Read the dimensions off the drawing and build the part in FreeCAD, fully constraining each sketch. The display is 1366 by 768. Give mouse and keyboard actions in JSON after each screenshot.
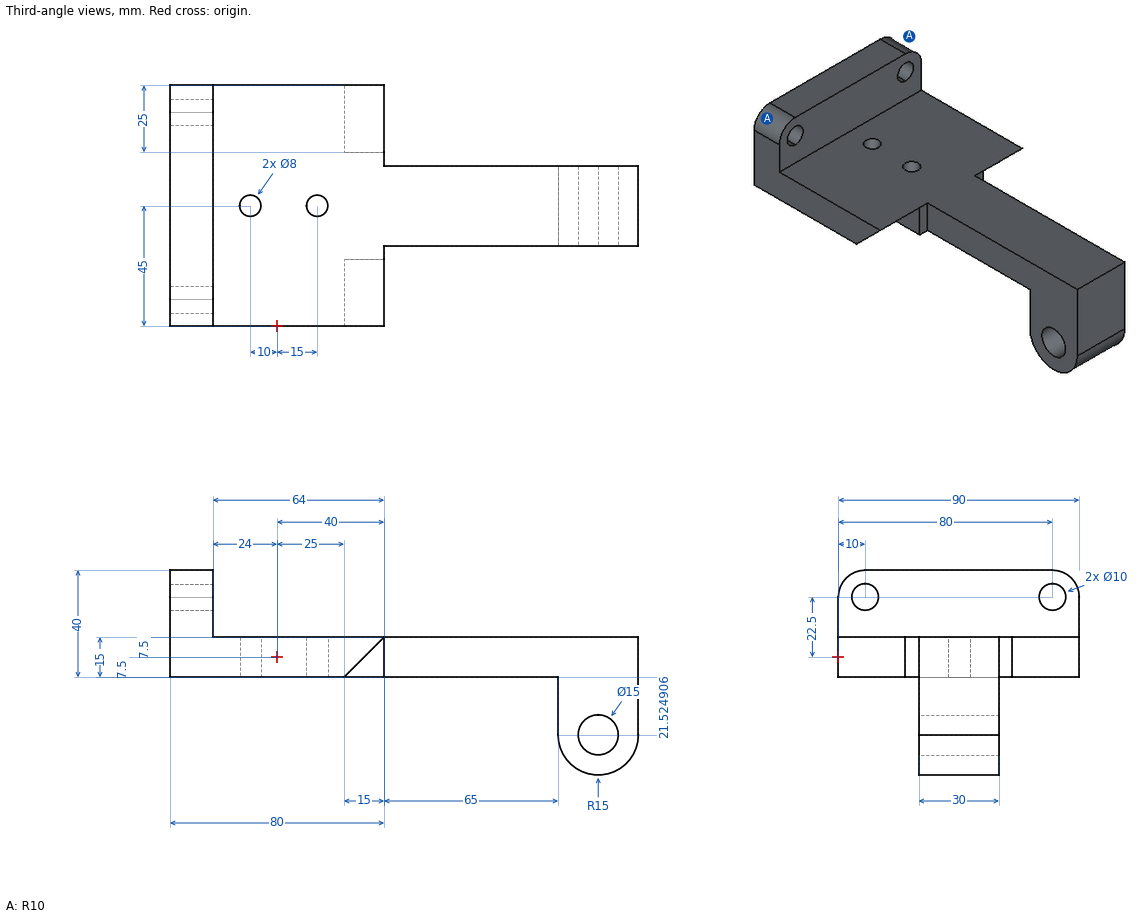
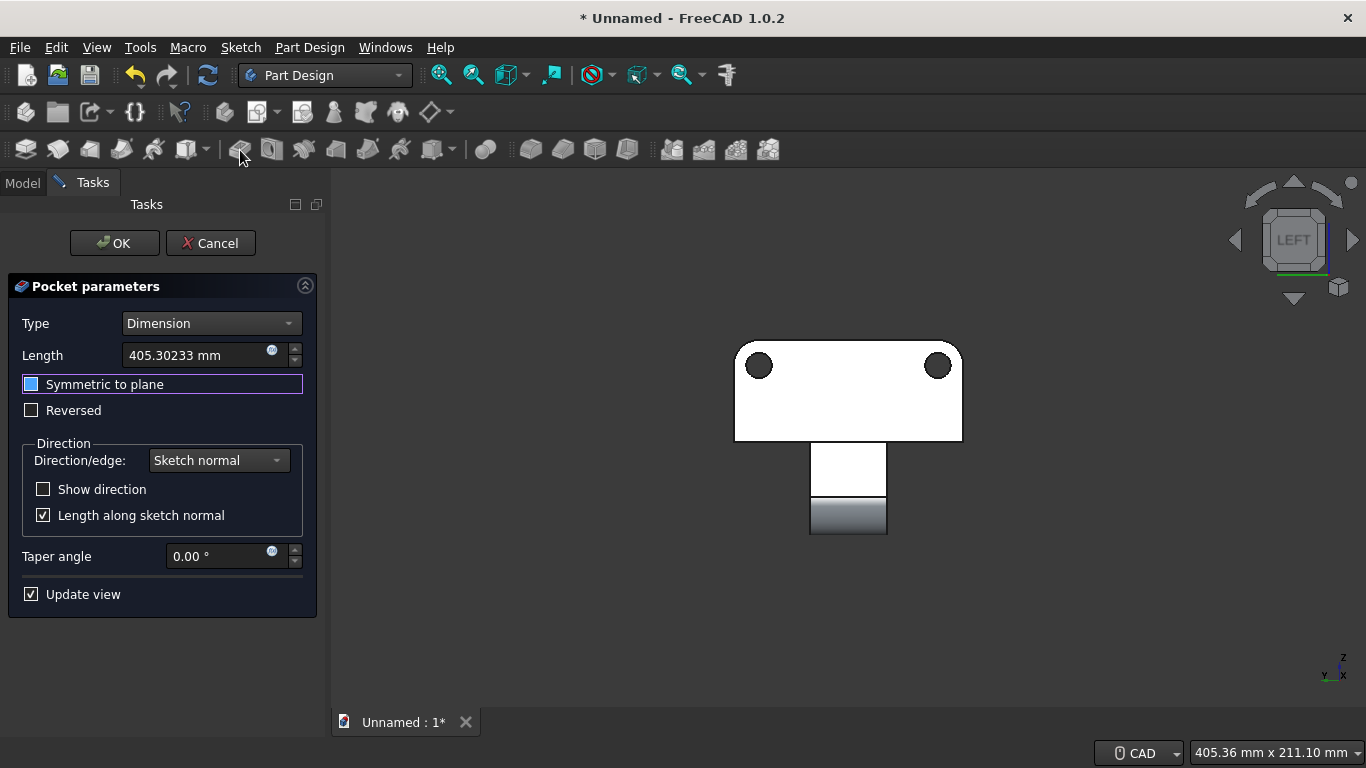
{"action": "left_click", "coordinate": [30, 384]}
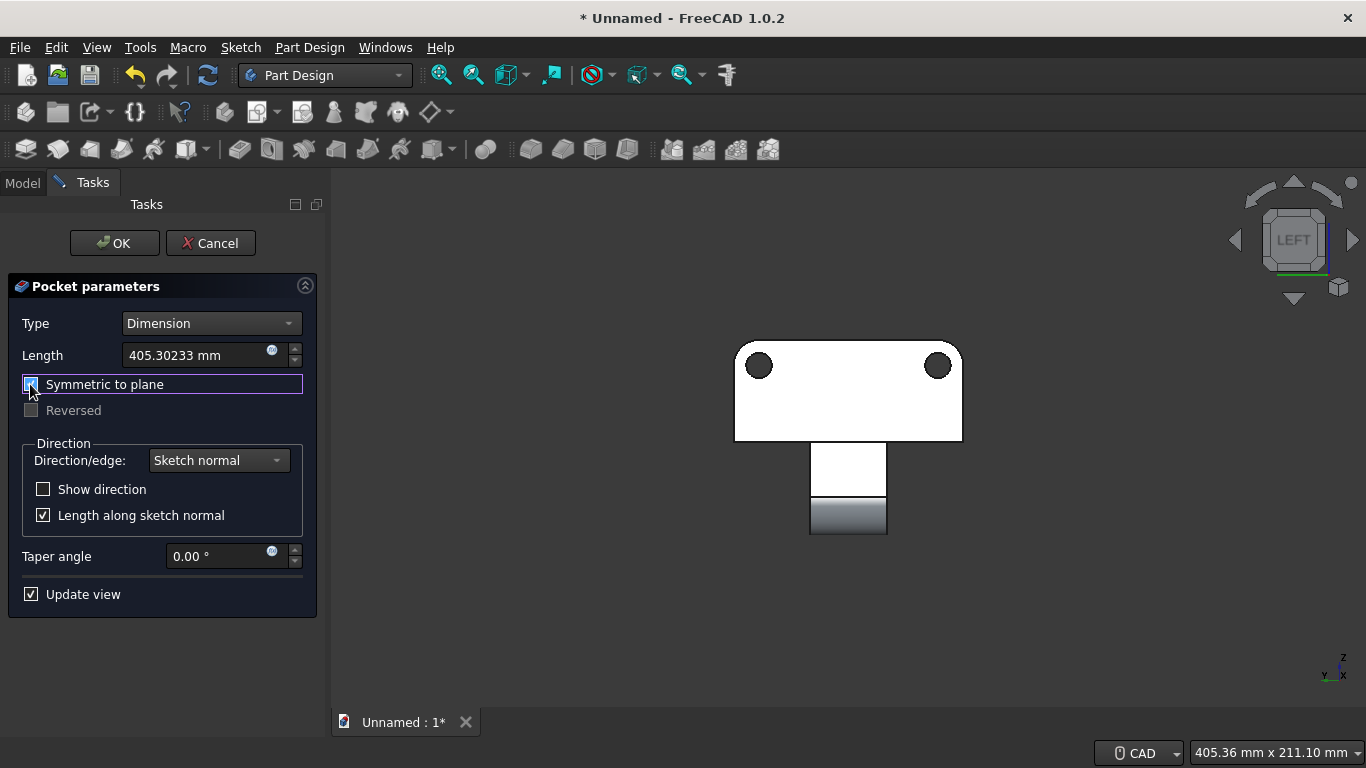
{"action": "left_click", "coordinate": [115, 243]}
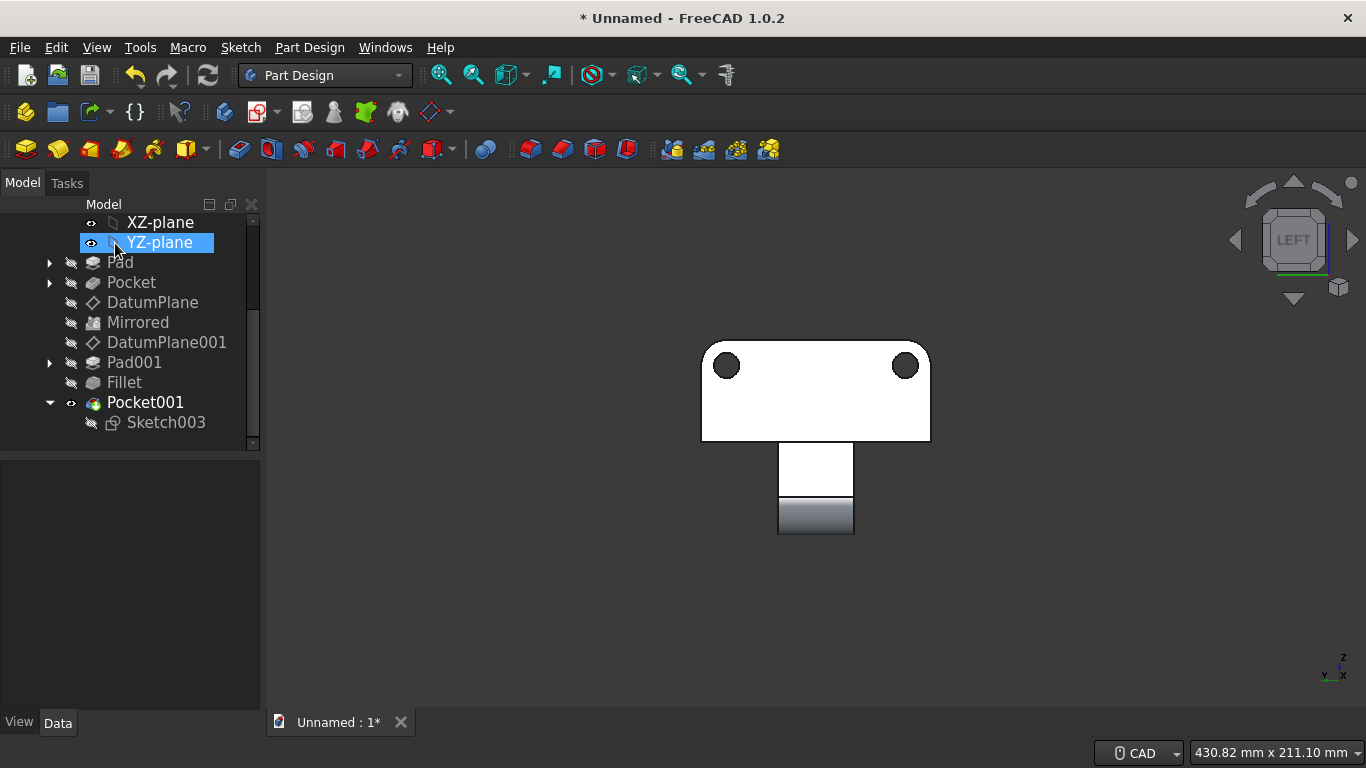
{"action": "left_click", "coordinate": [442, 76]}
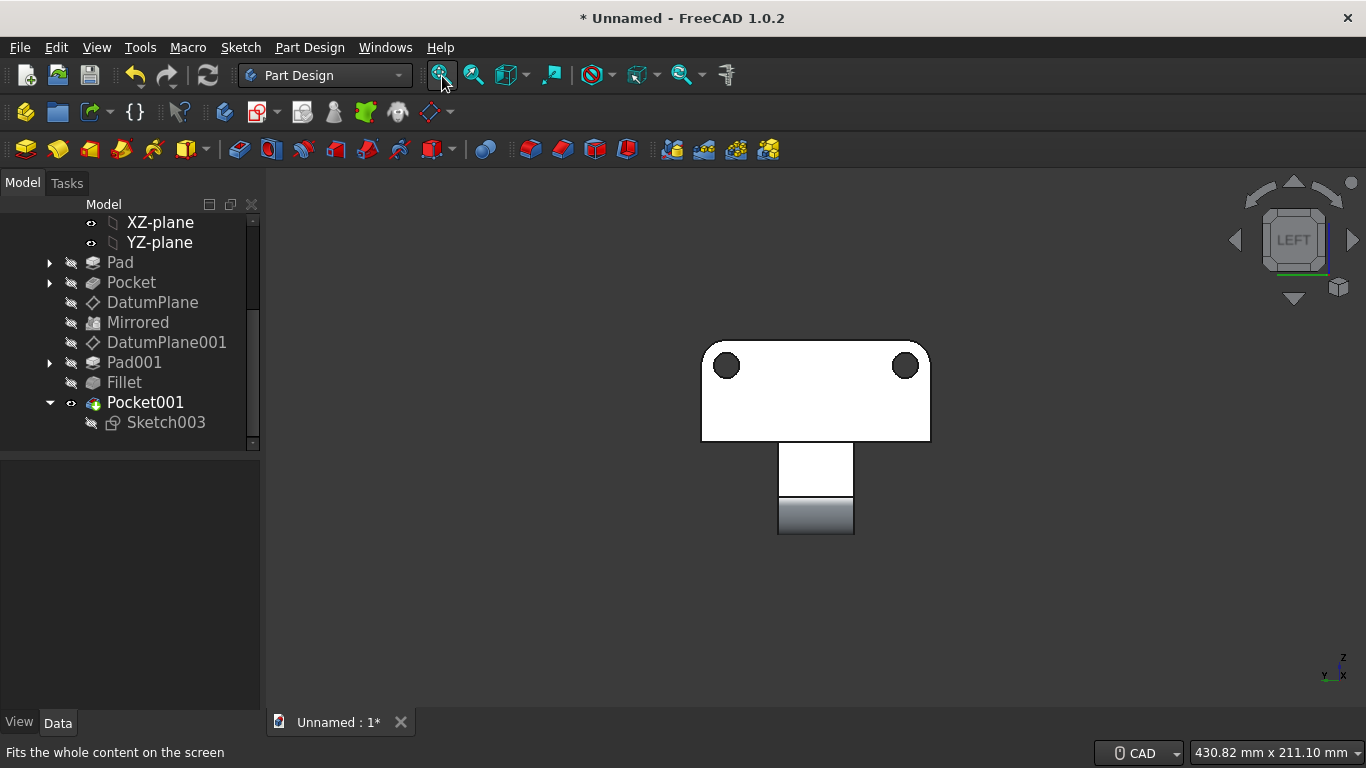
{"action": "key", "text": "5"}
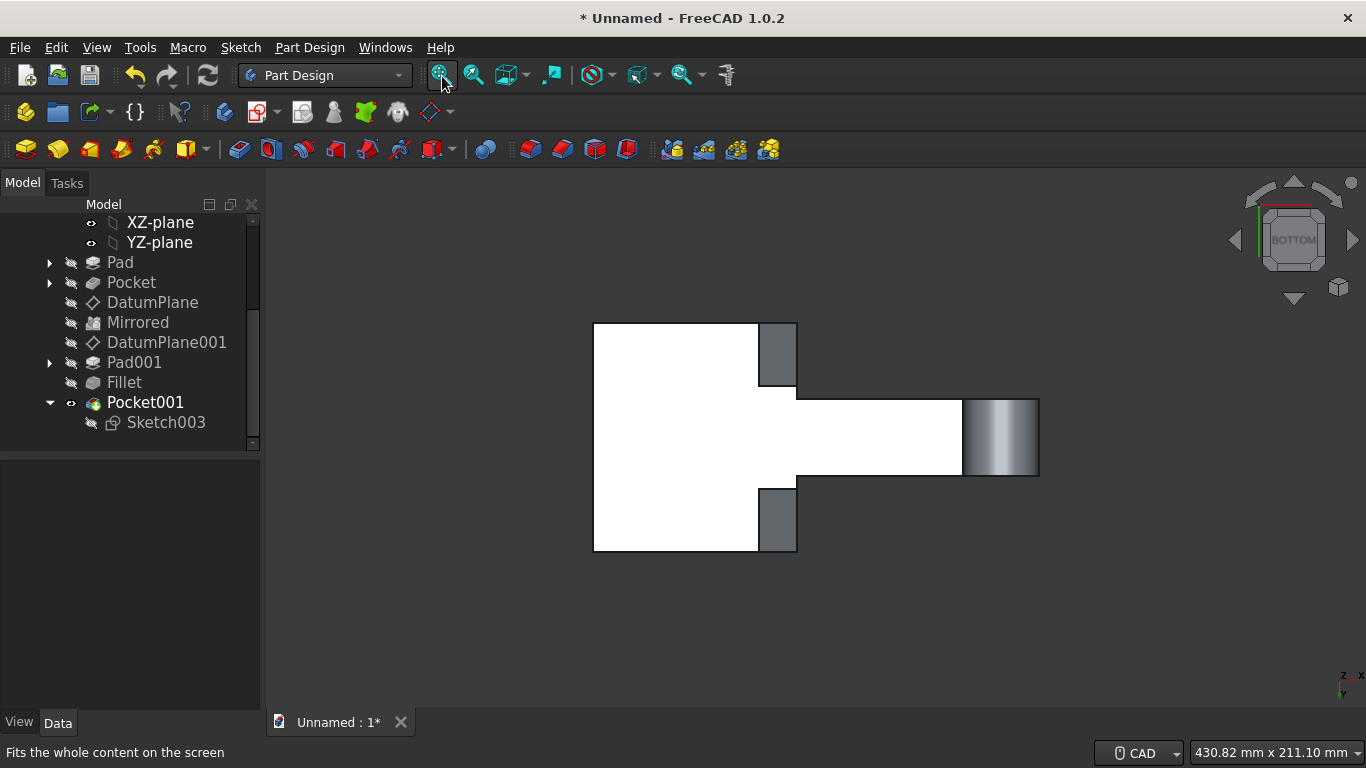
{"action": "left_click", "coordinate": [442, 76]}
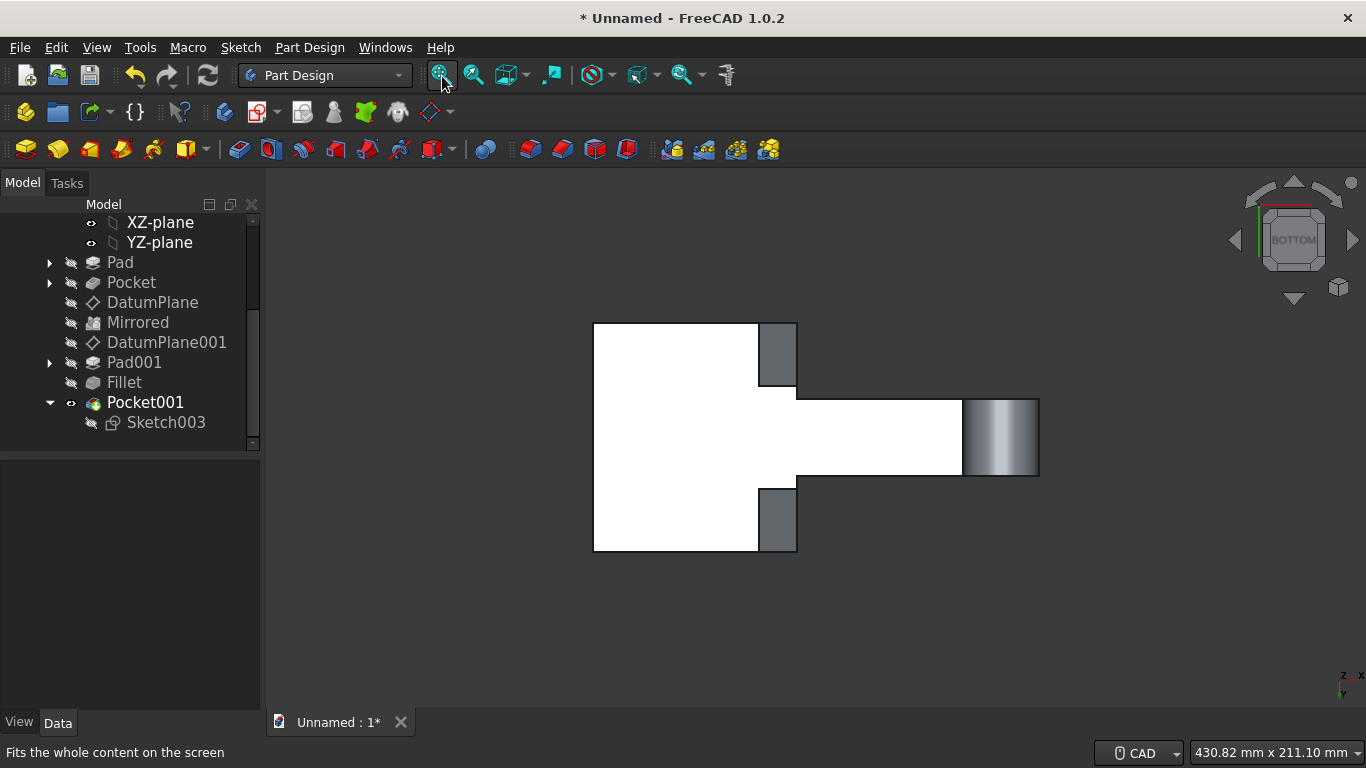
{"action": "left_click", "coordinate": [672, 469]}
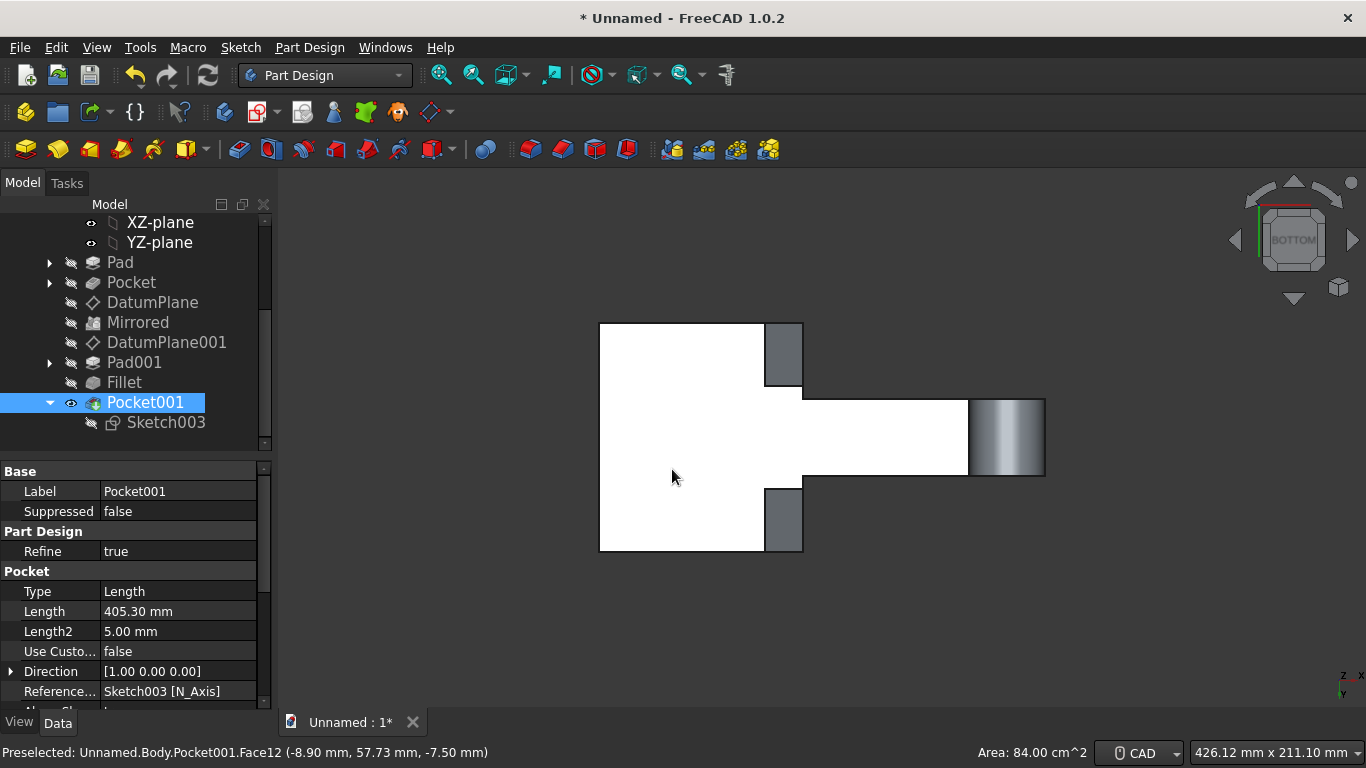
{"action": "left_click", "coordinate": [258, 112]}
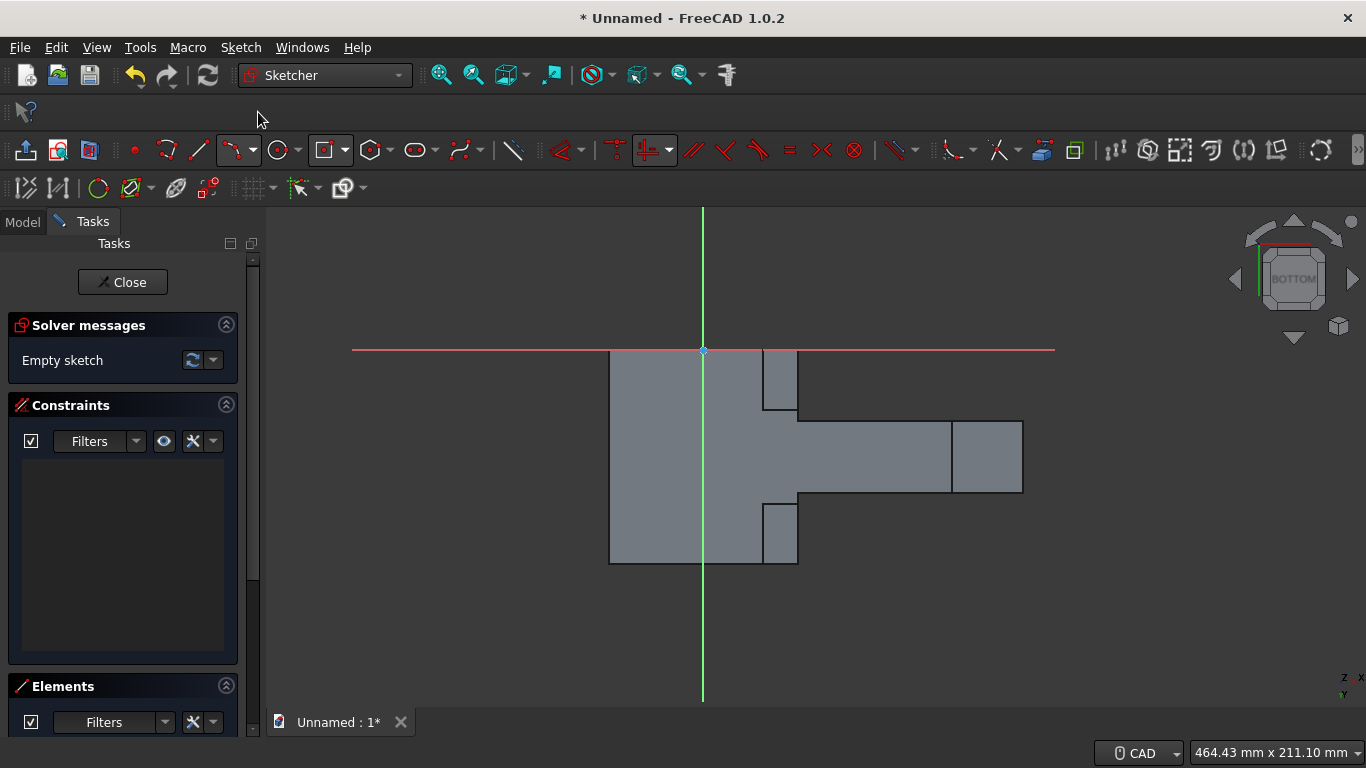
{"action": "left_click", "coordinate": [90, 150]}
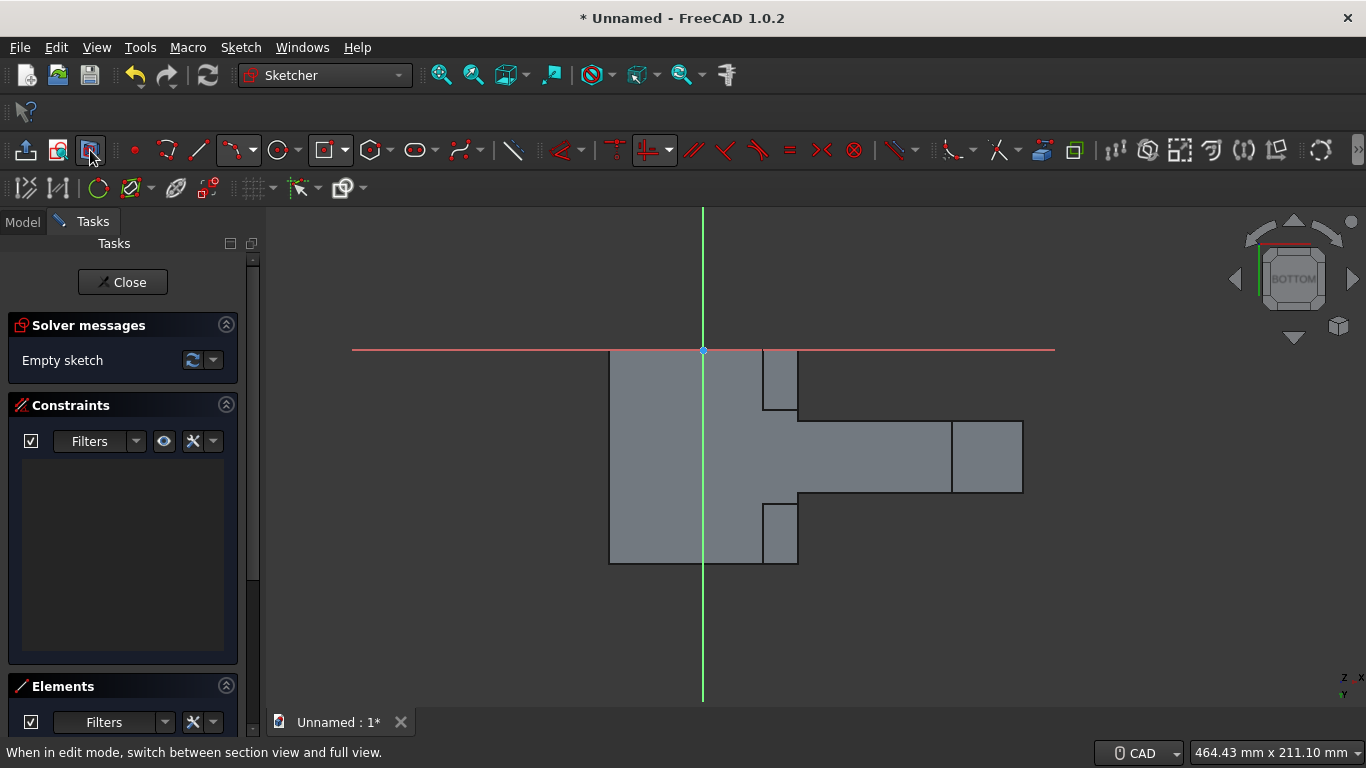
{"action": "scroll", "coordinate": [687, 380], "scroll_direction": "up", "scroll_amount": 5}